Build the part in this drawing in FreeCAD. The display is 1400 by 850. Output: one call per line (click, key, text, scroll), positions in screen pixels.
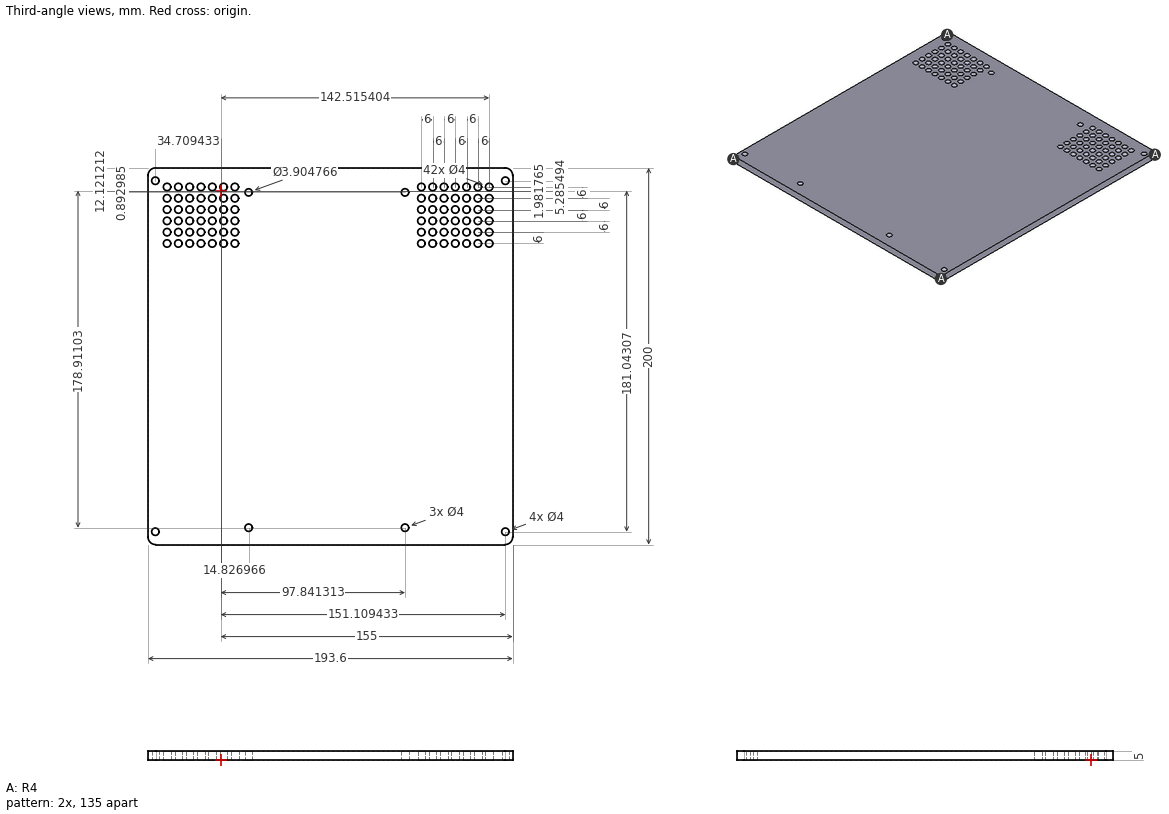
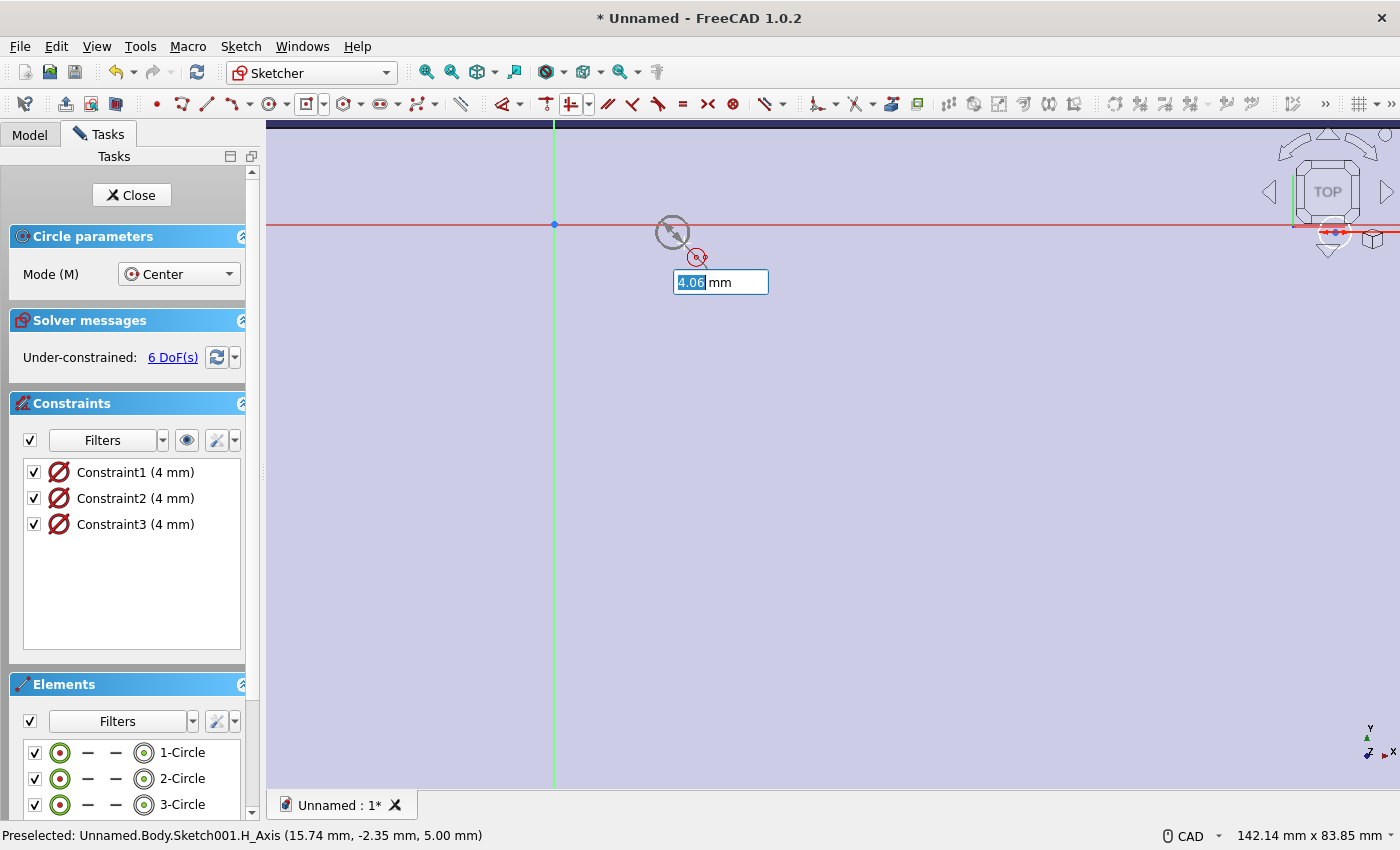
text(3.904766)
key(Return)
key(Escape)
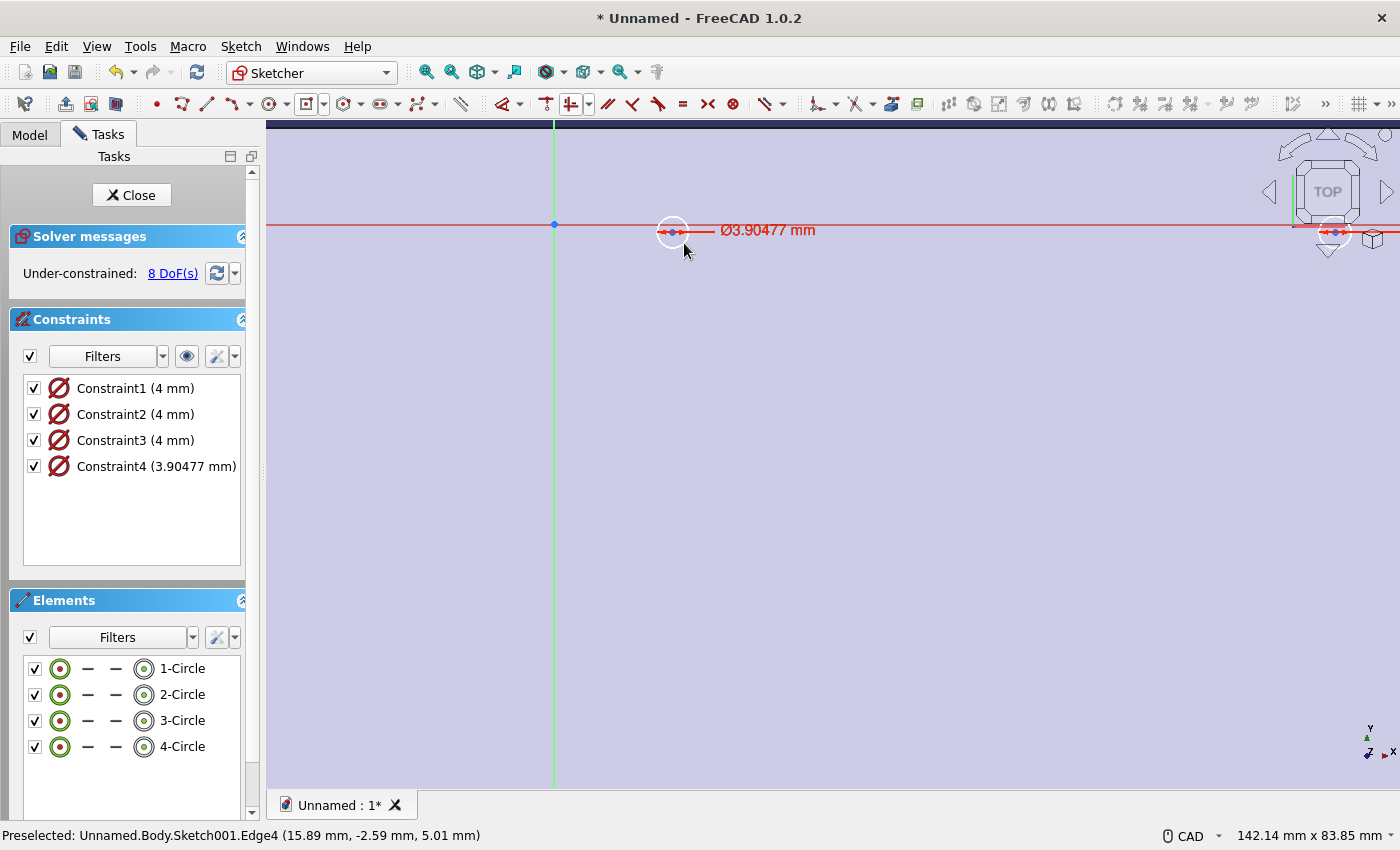
click(502, 104)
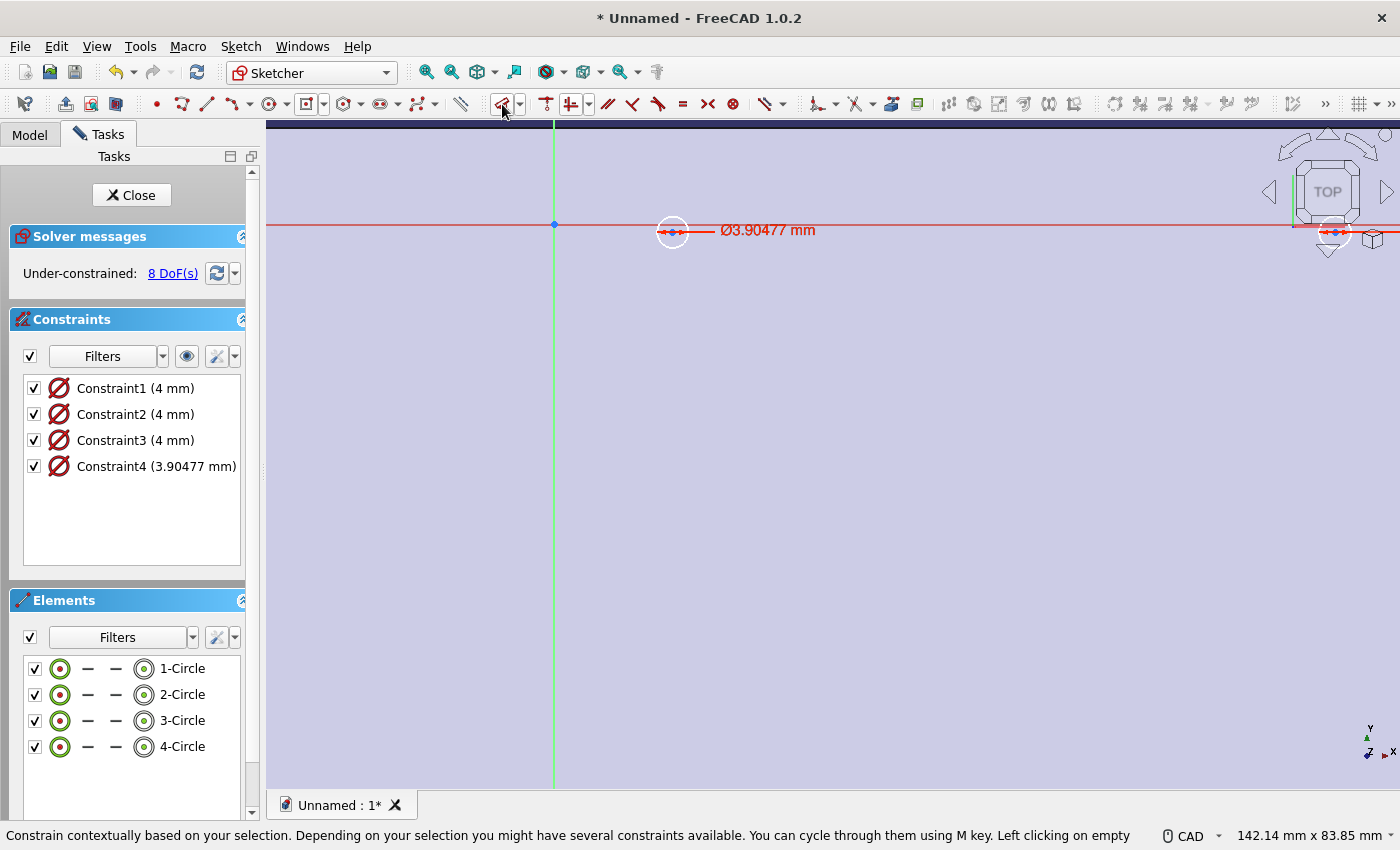
scroll(683, 244, down, 6)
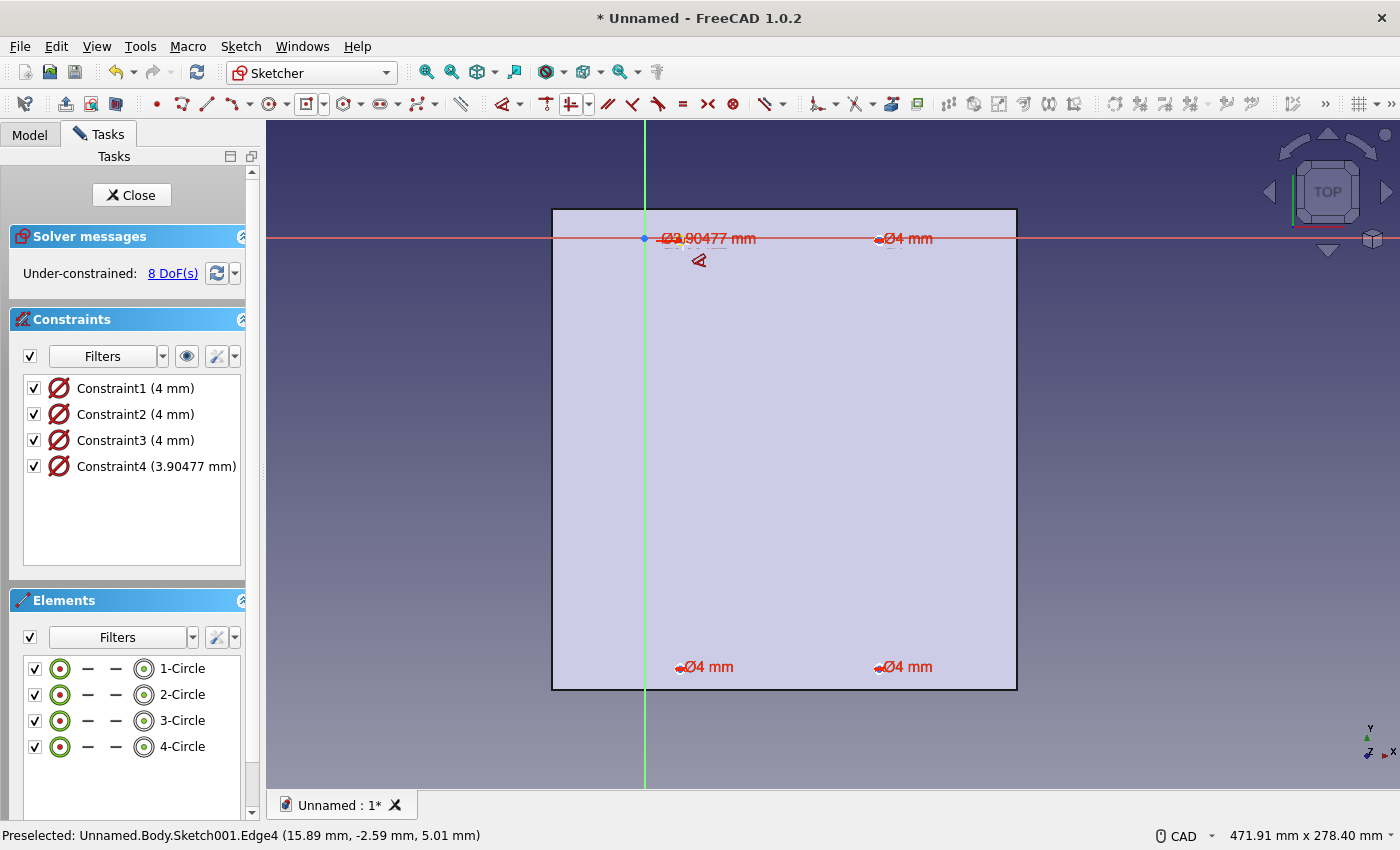
scroll(880, 241, up, 15)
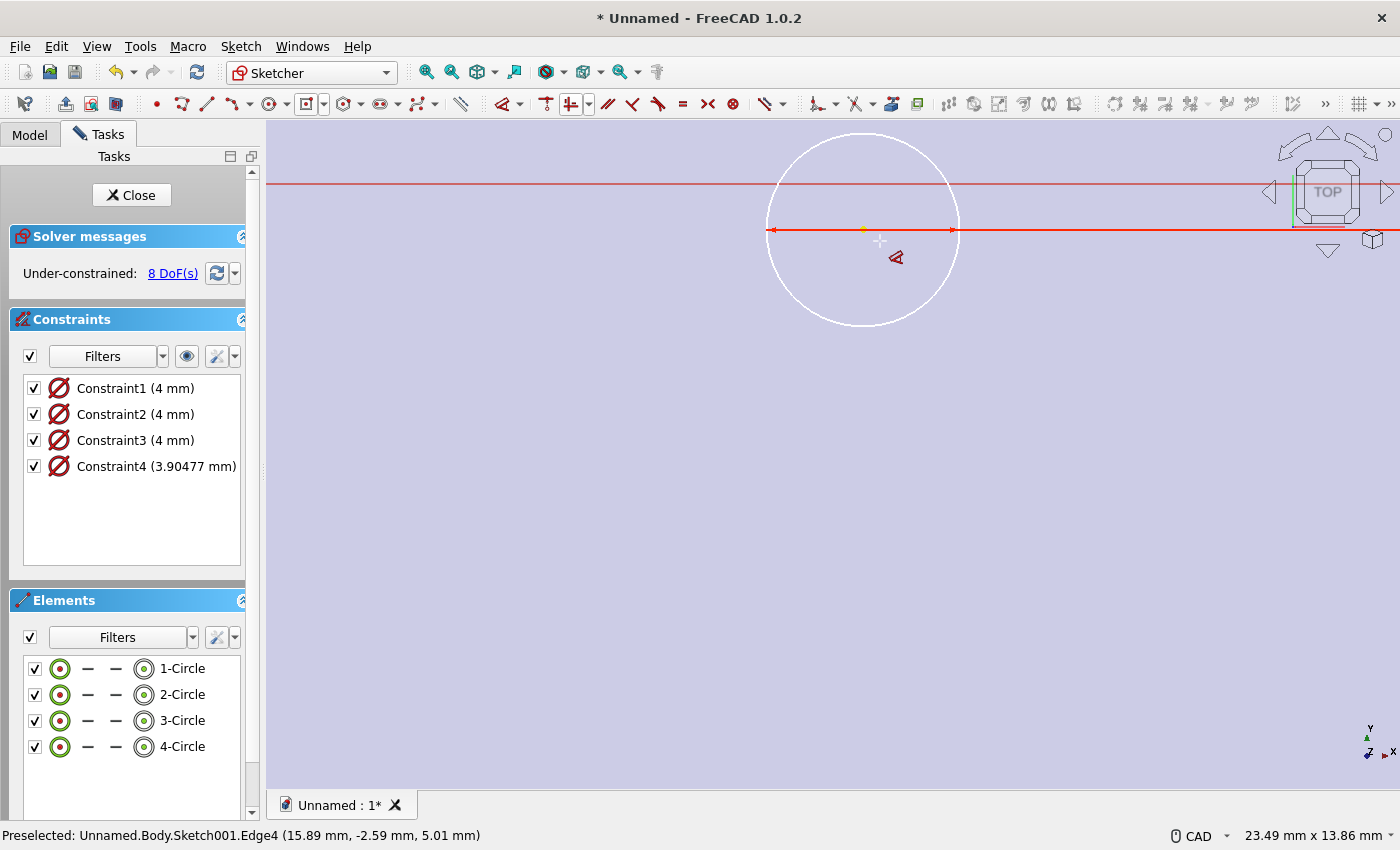
click(863, 230)
click(897, 207)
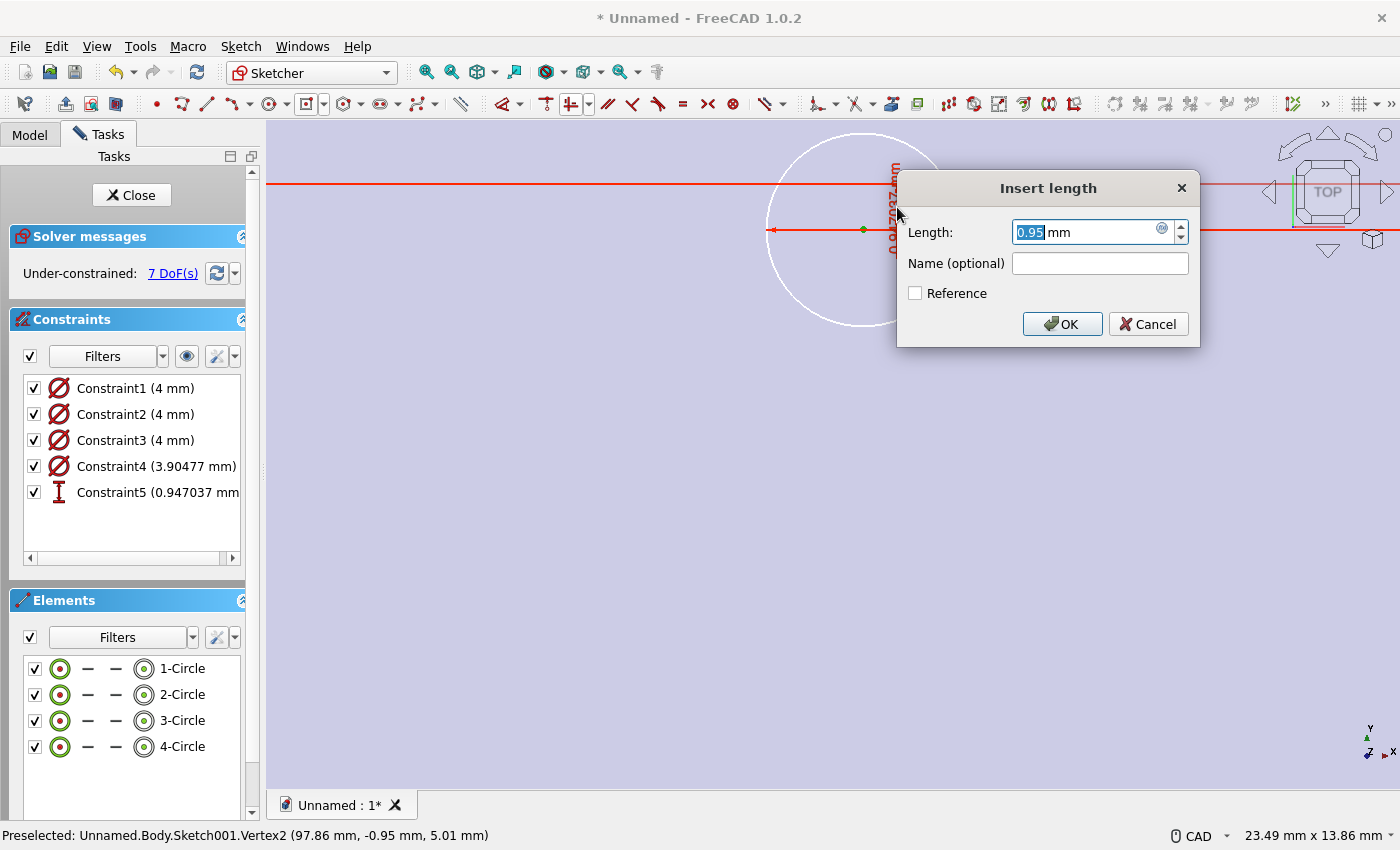
text(0.892985)
key(Return)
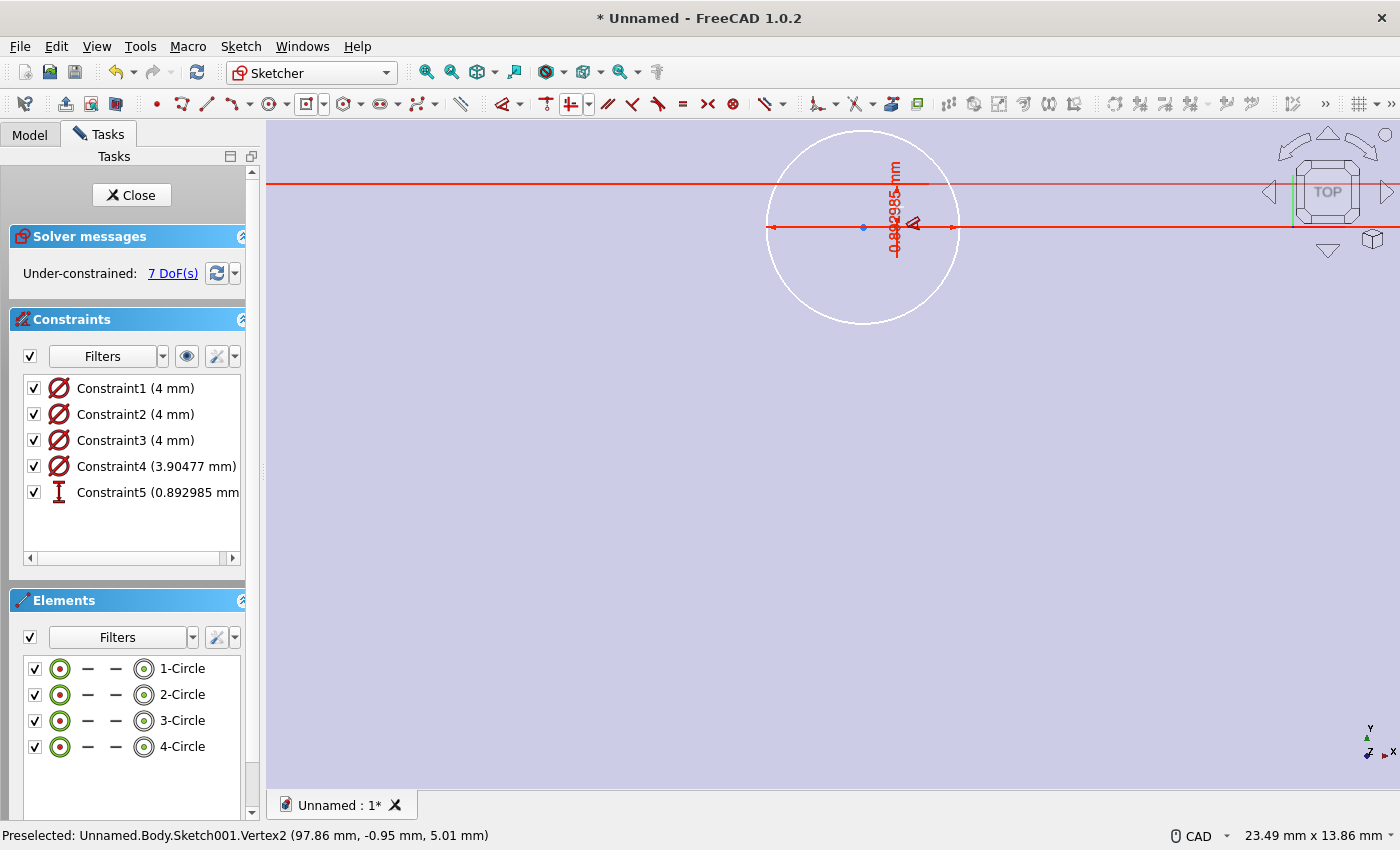
scroll(881, 241, down, 15)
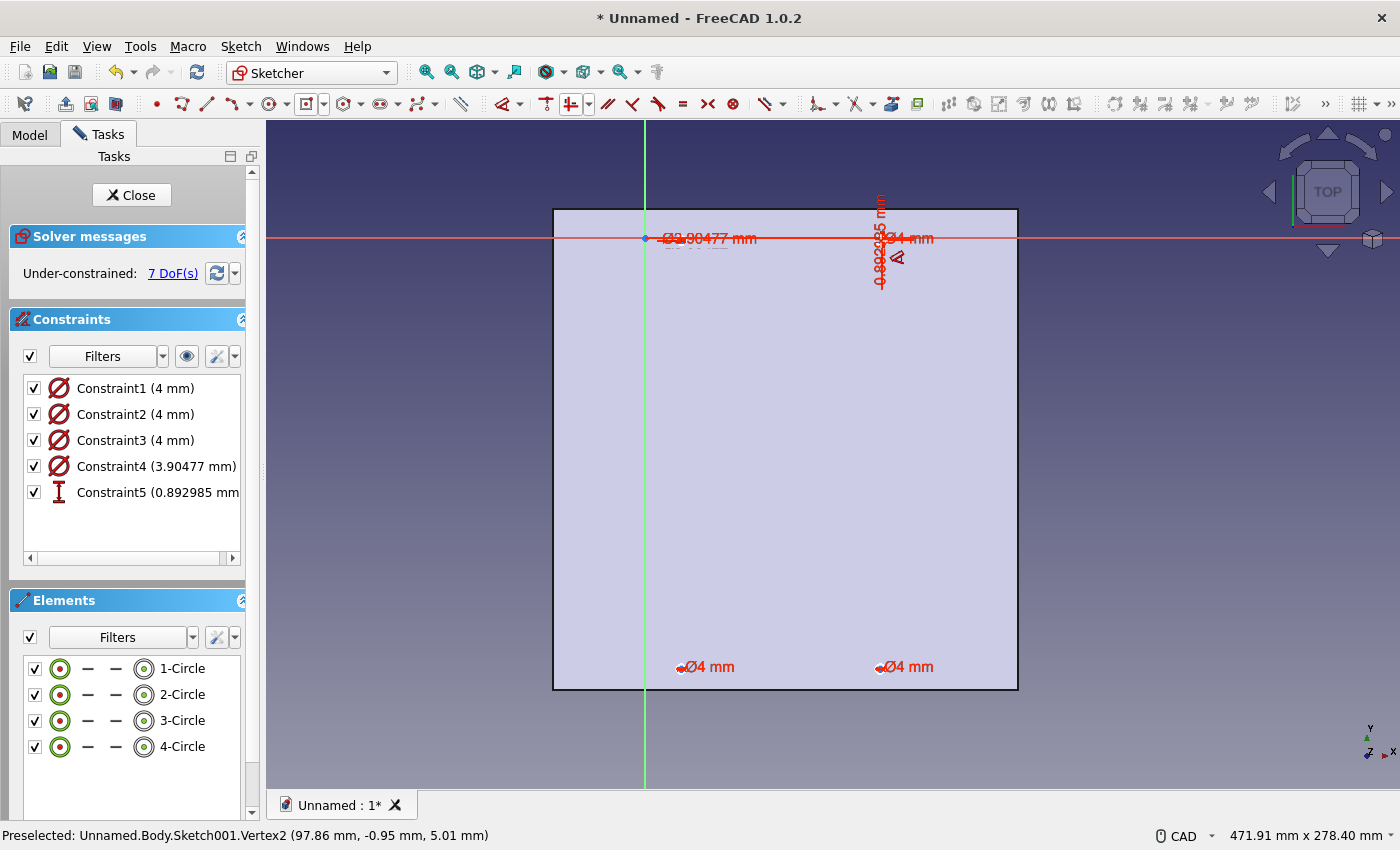
scroll(681, 241, up, 15)